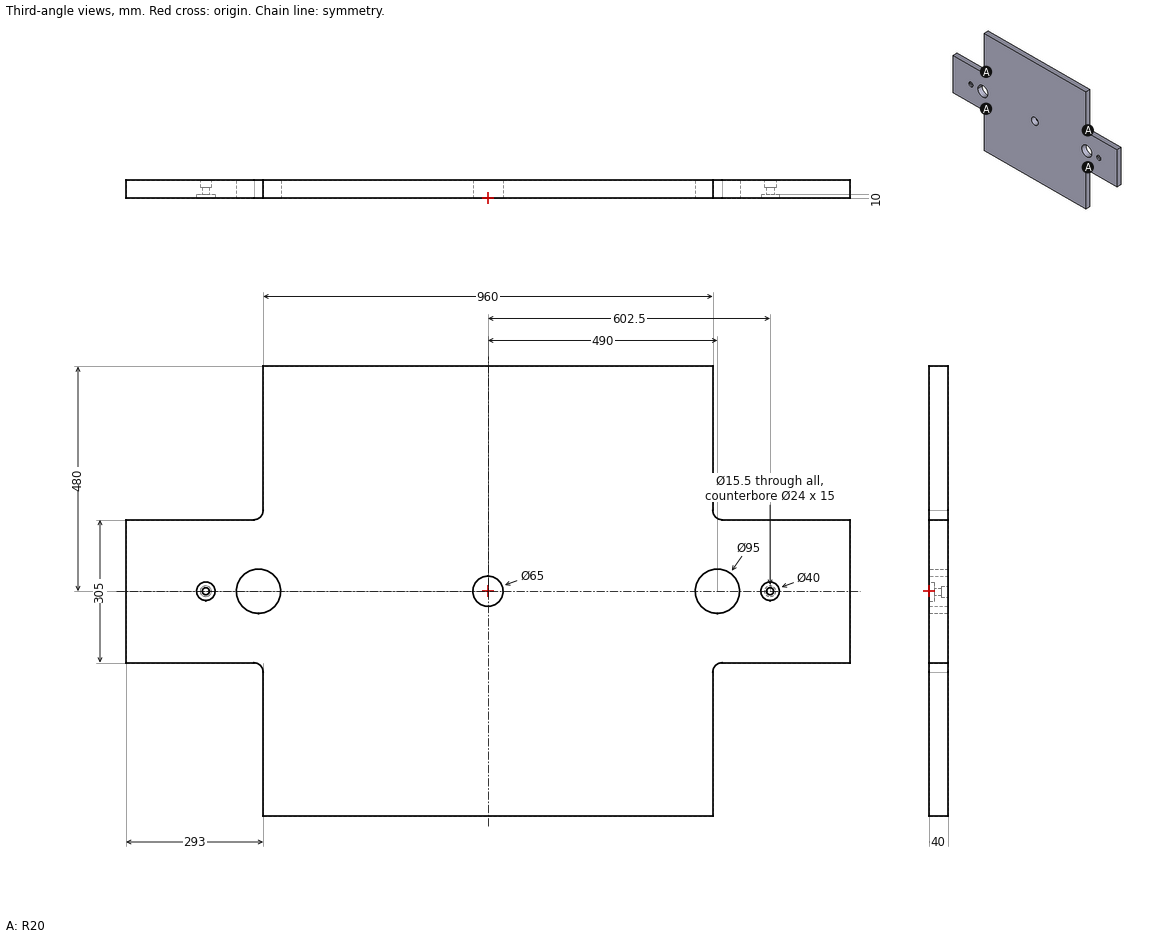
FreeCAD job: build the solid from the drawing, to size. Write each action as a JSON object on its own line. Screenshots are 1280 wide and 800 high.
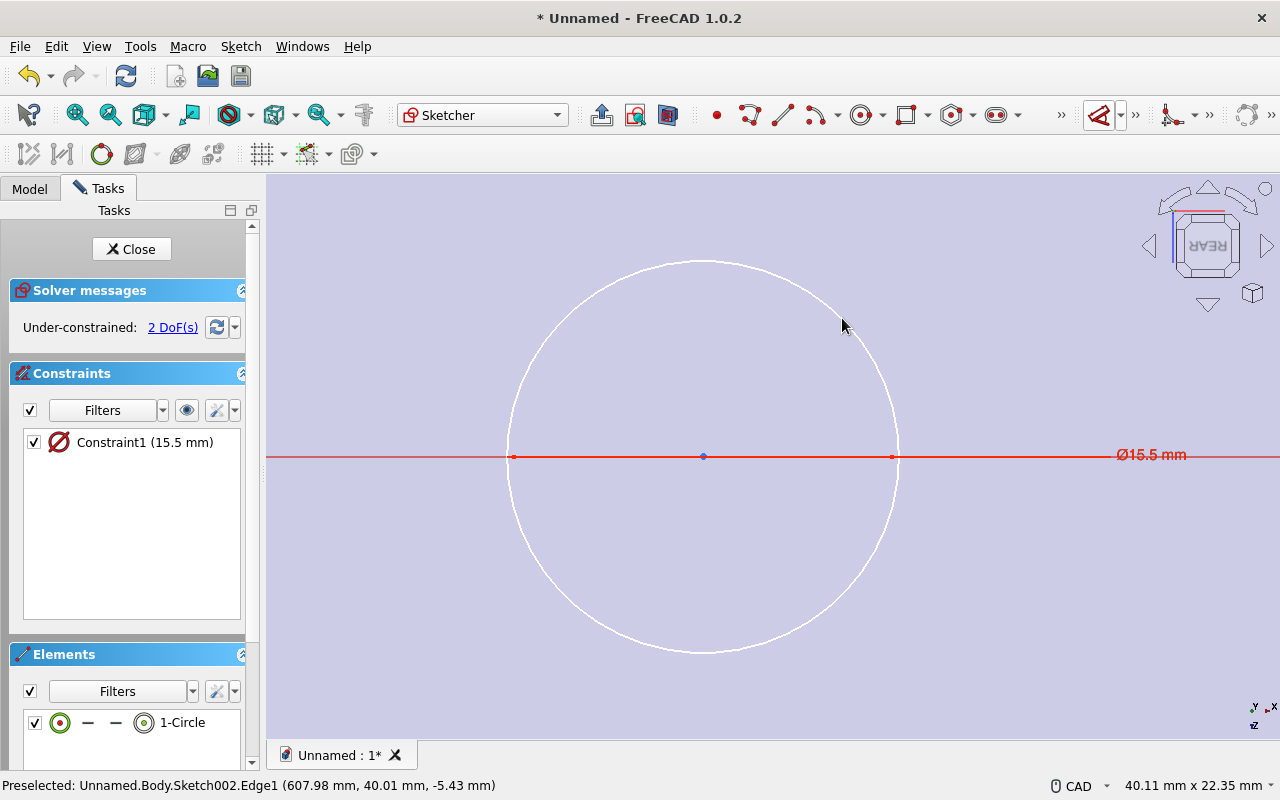
{"action": "left_click", "coordinate": [703, 457]}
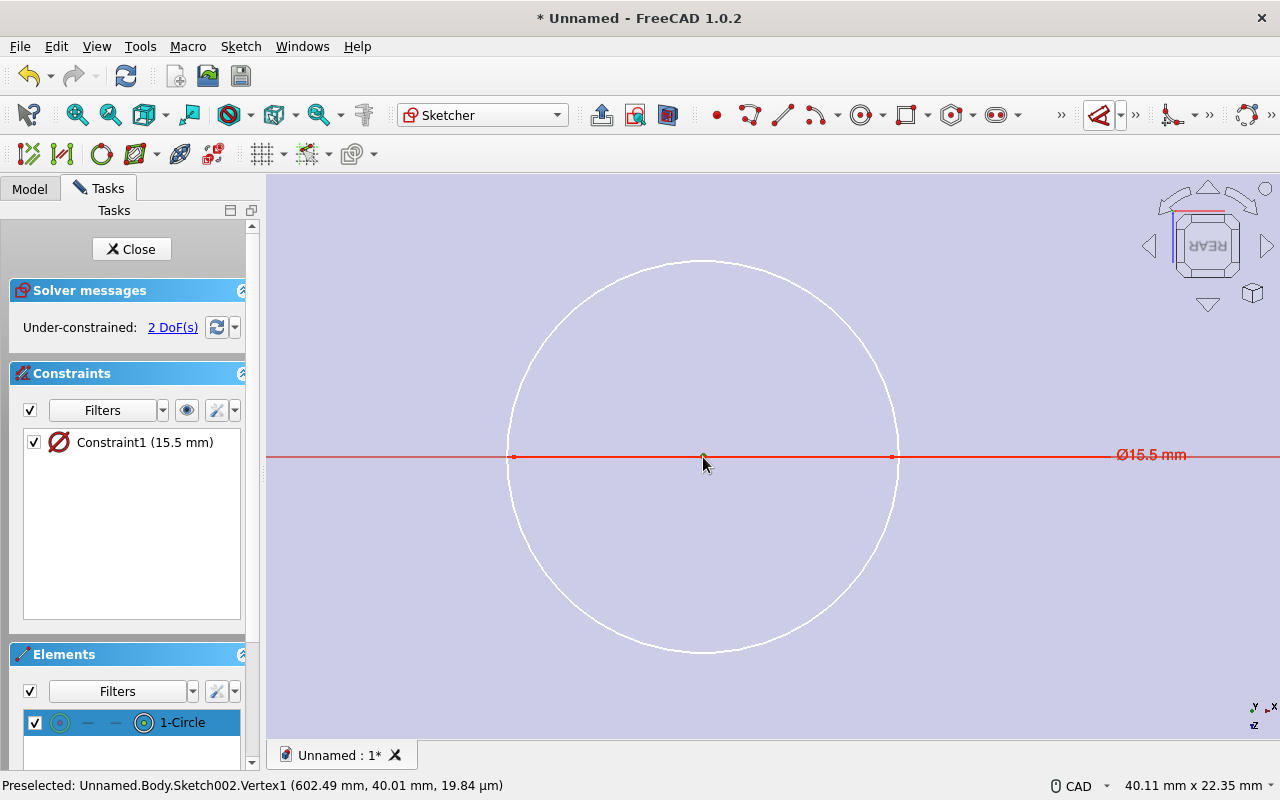
{"action": "left_click", "coordinate": [353, 456]}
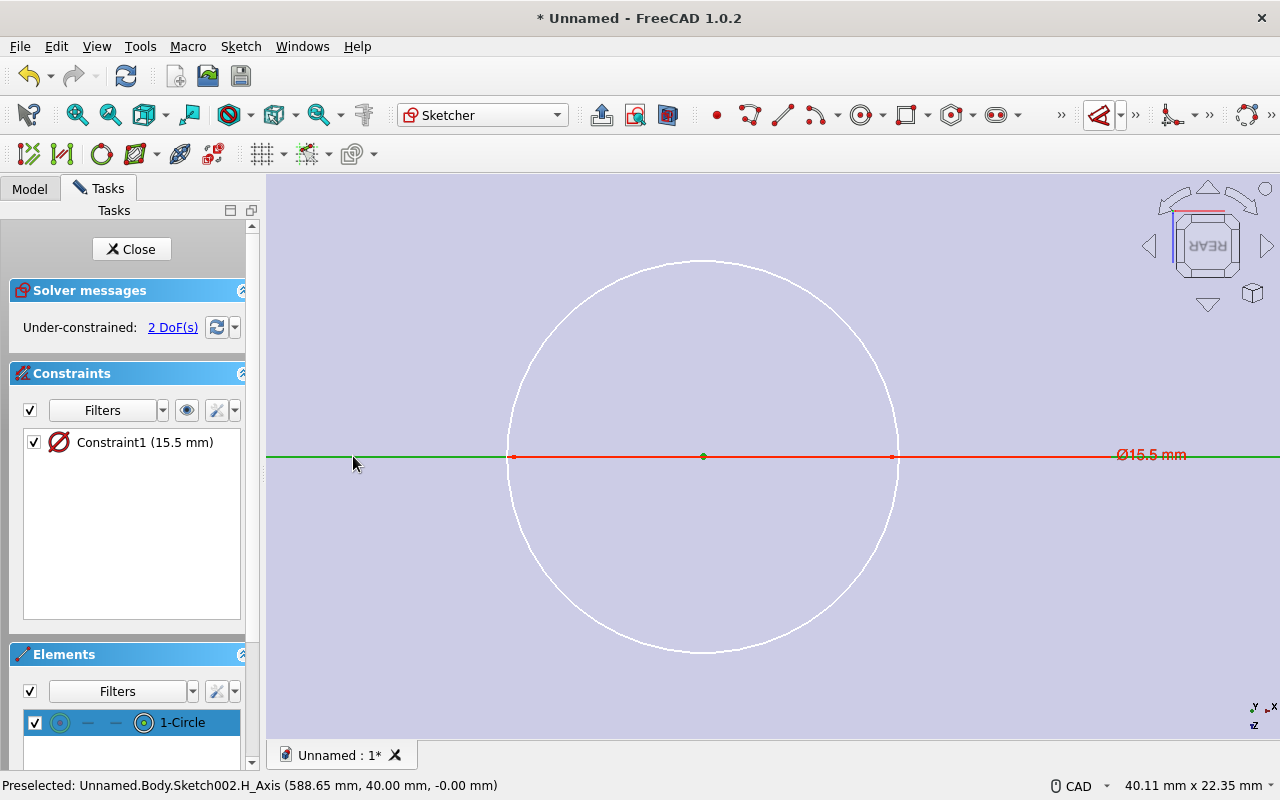
{"action": "key", "text": "c"}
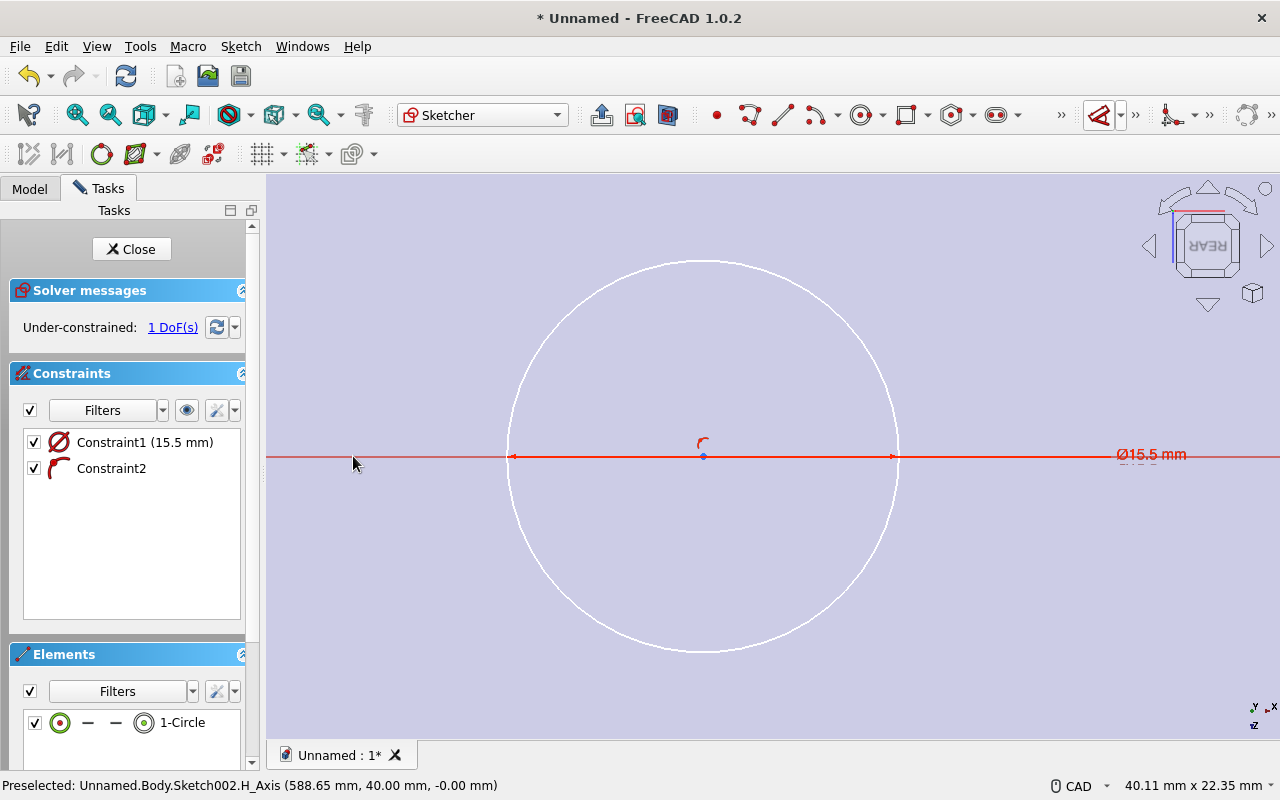
{"action": "left_click", "coordinate": [703, 456]}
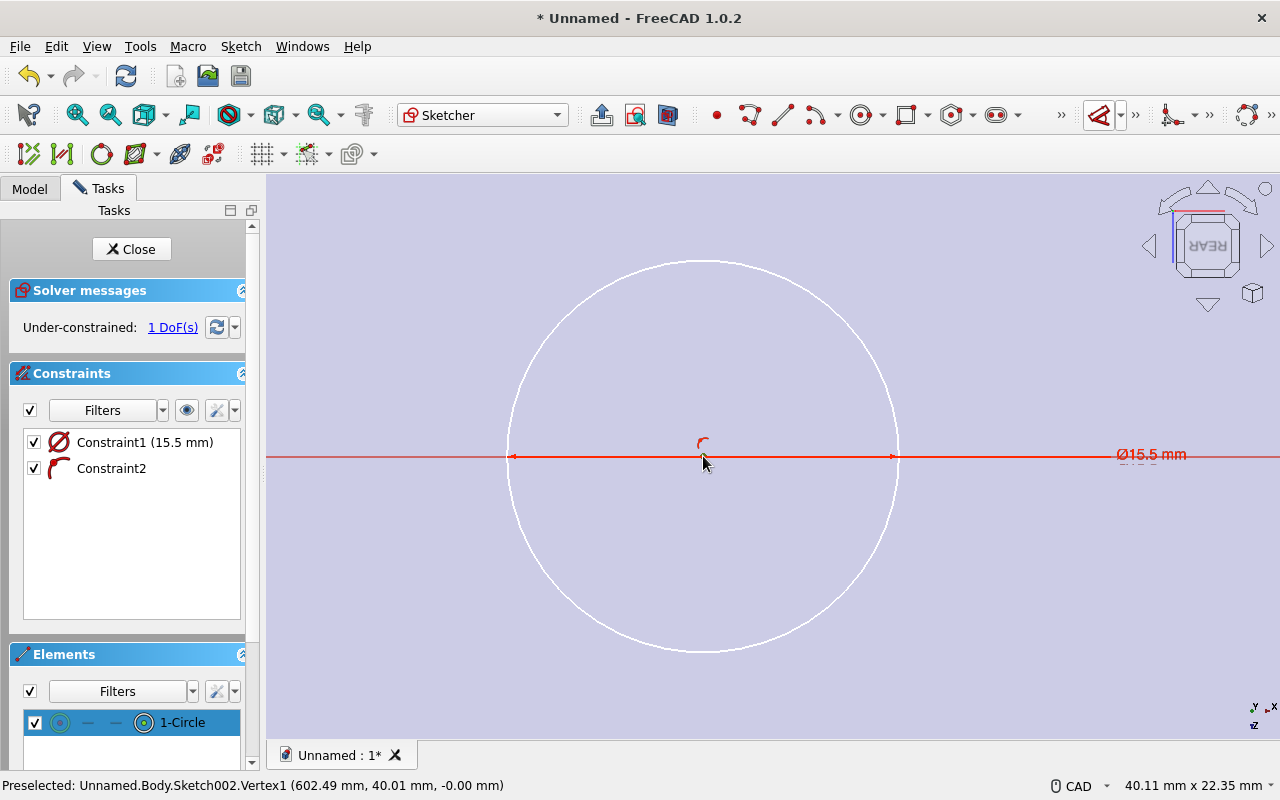
{"action": "key", "text": "l"}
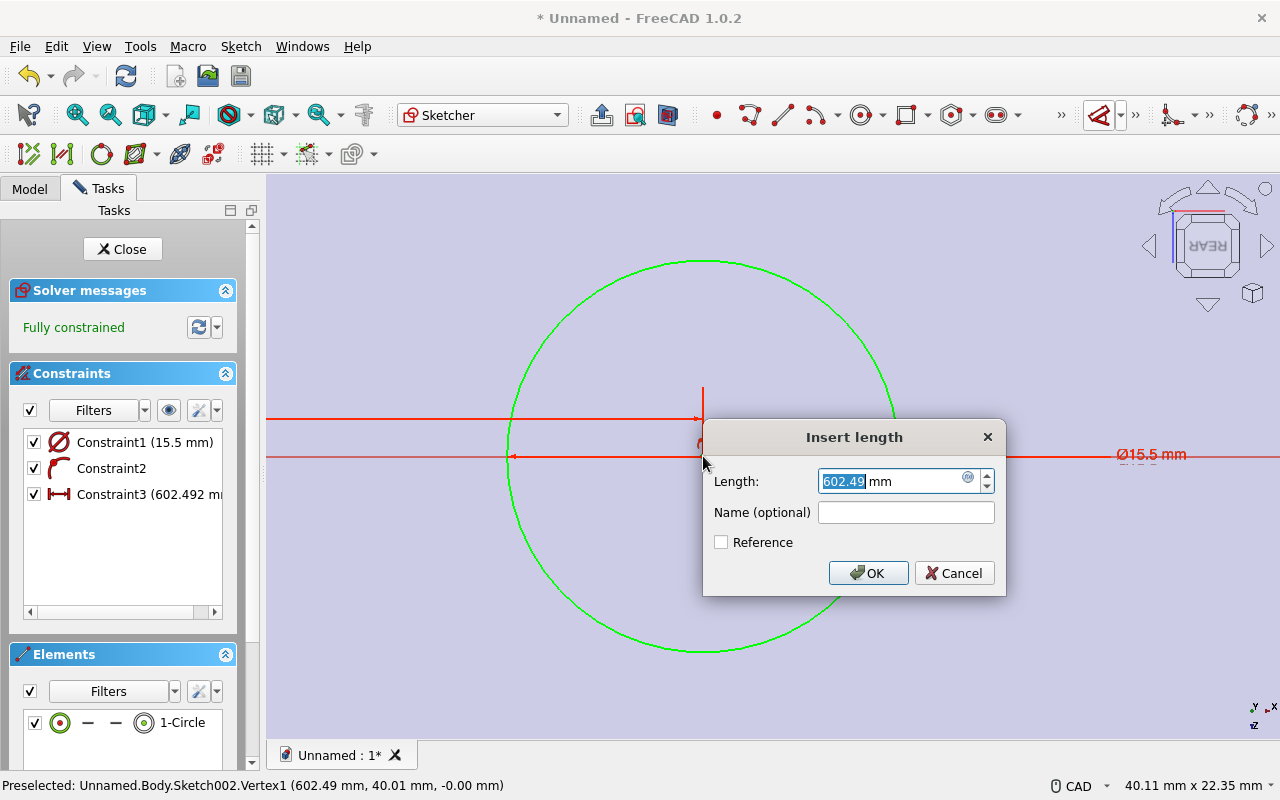
{"action": "type", "text": "602.5"}
{"action": "key", "text": "Return"}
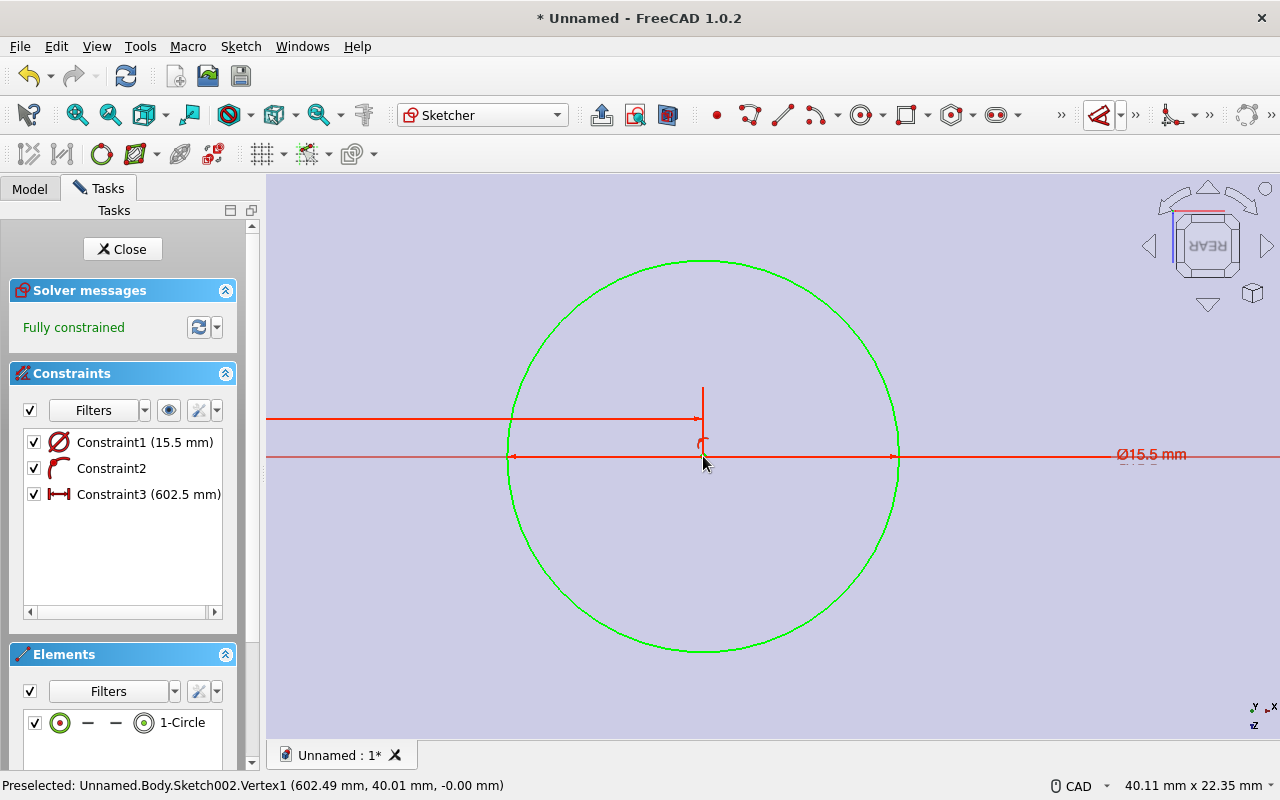
{"action": "left_click", "coordinate": [123, 249]}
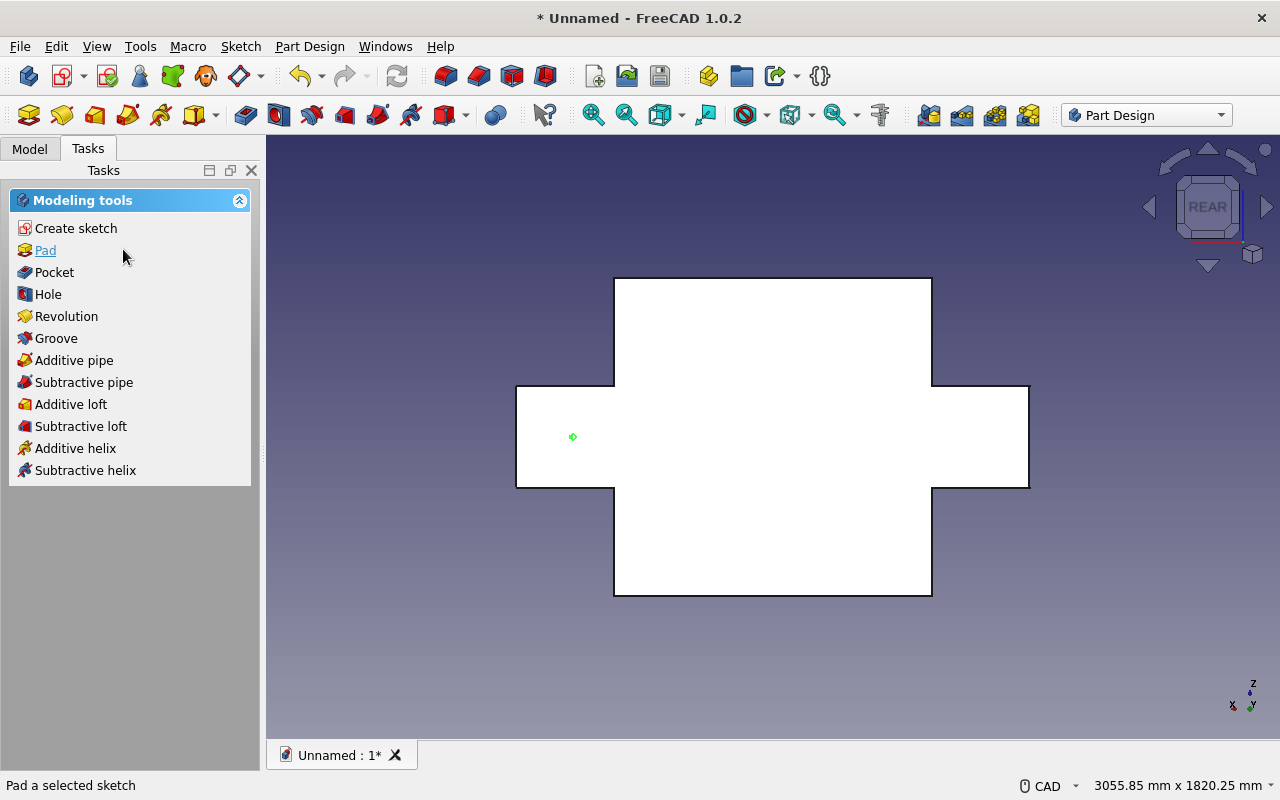
{"action": "left_click", "coordinate": [279, 116]}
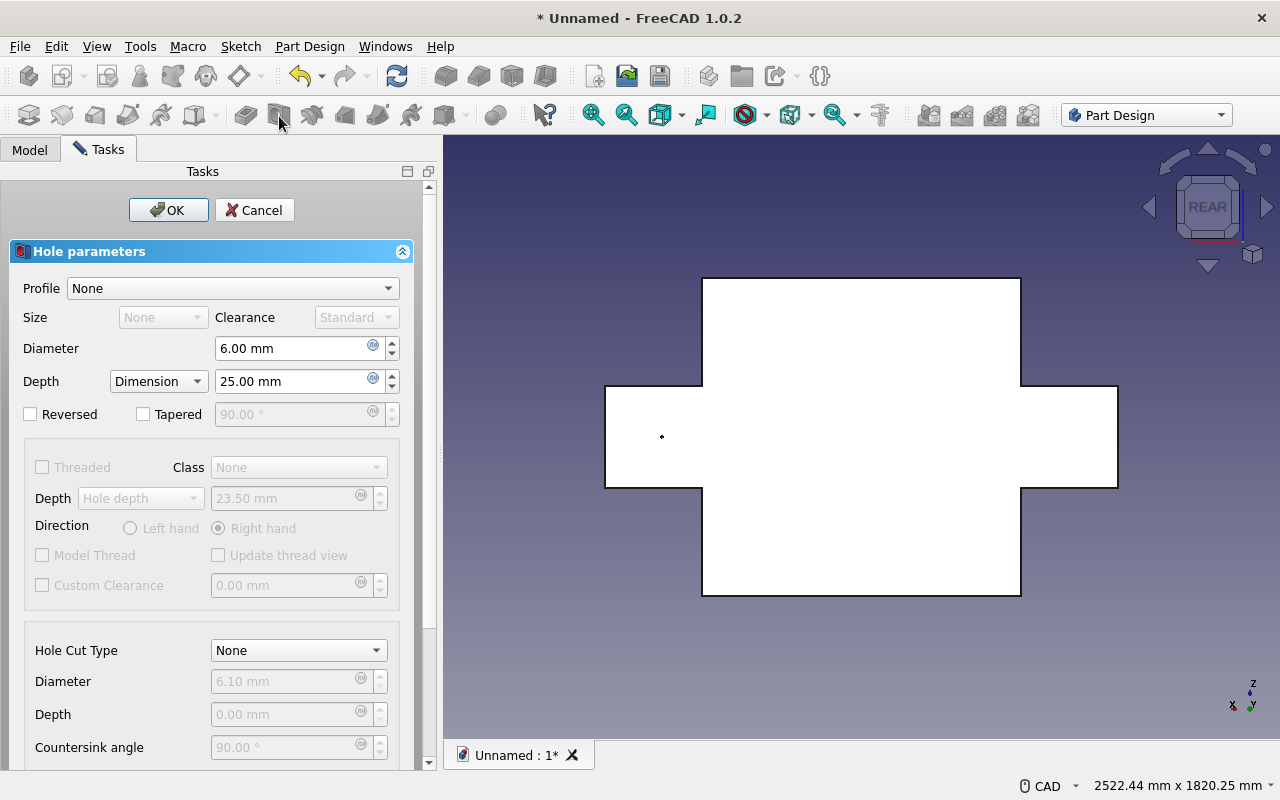
{"action": "triple_click", "coordinate": [300, 348]}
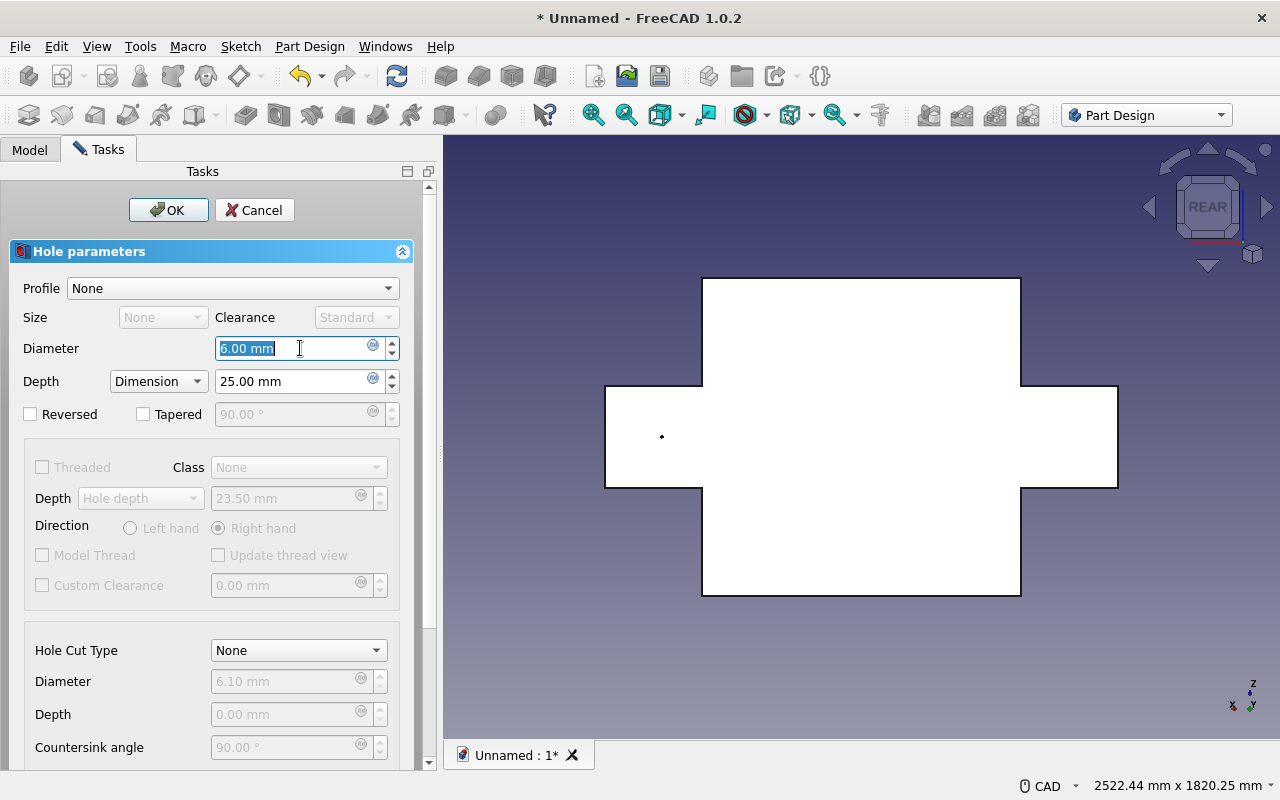
{"action": "type", "text": "15.5"}
{"action": "key", "text": "Tab"}